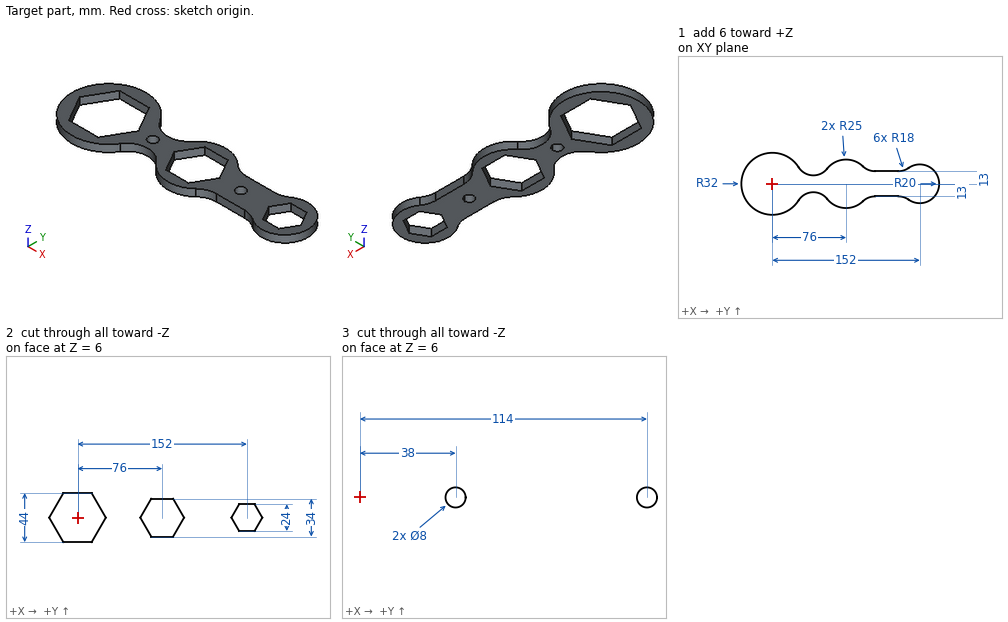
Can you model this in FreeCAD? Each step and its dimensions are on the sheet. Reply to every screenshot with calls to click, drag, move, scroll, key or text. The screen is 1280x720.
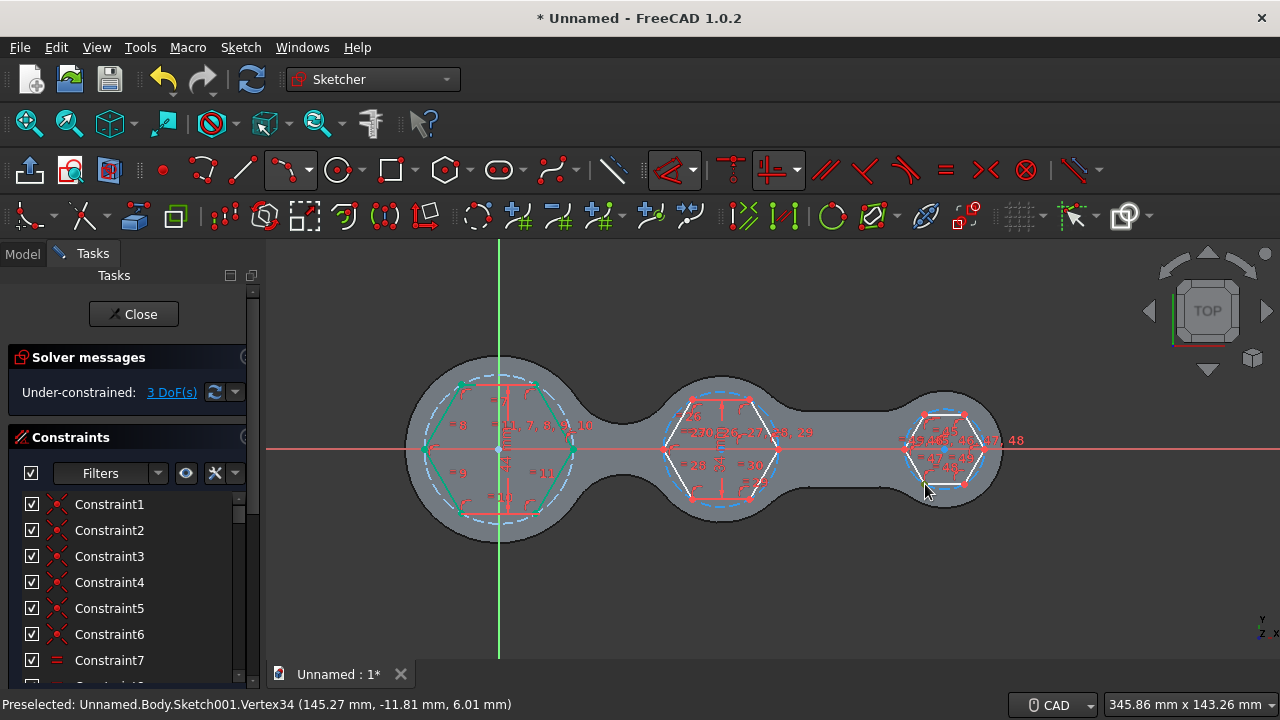
click(965, 415)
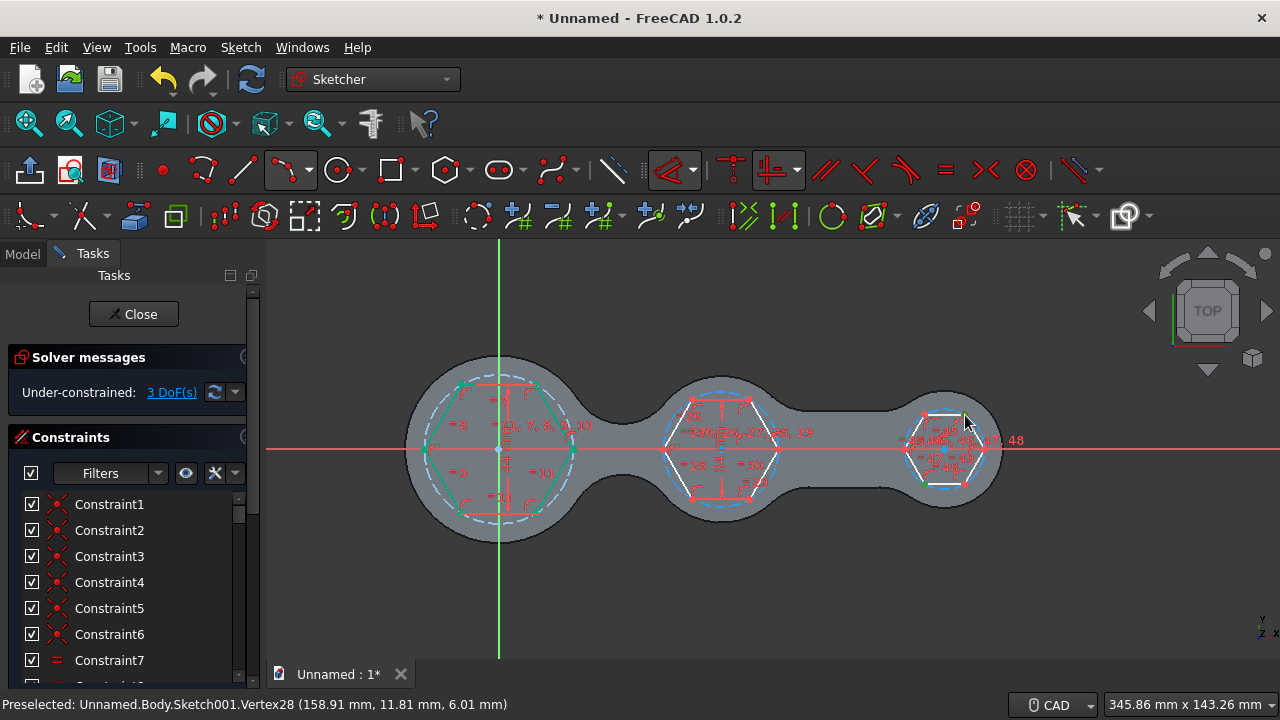
click(696, 170)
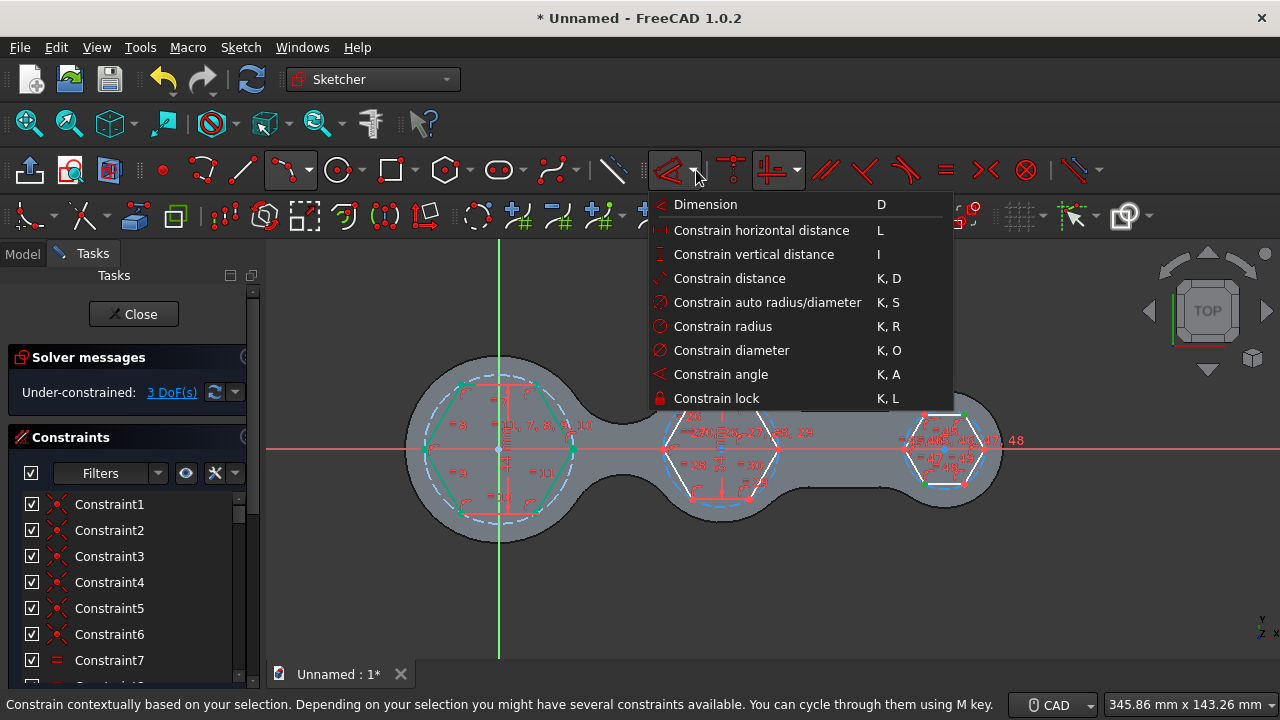
click(801, 254)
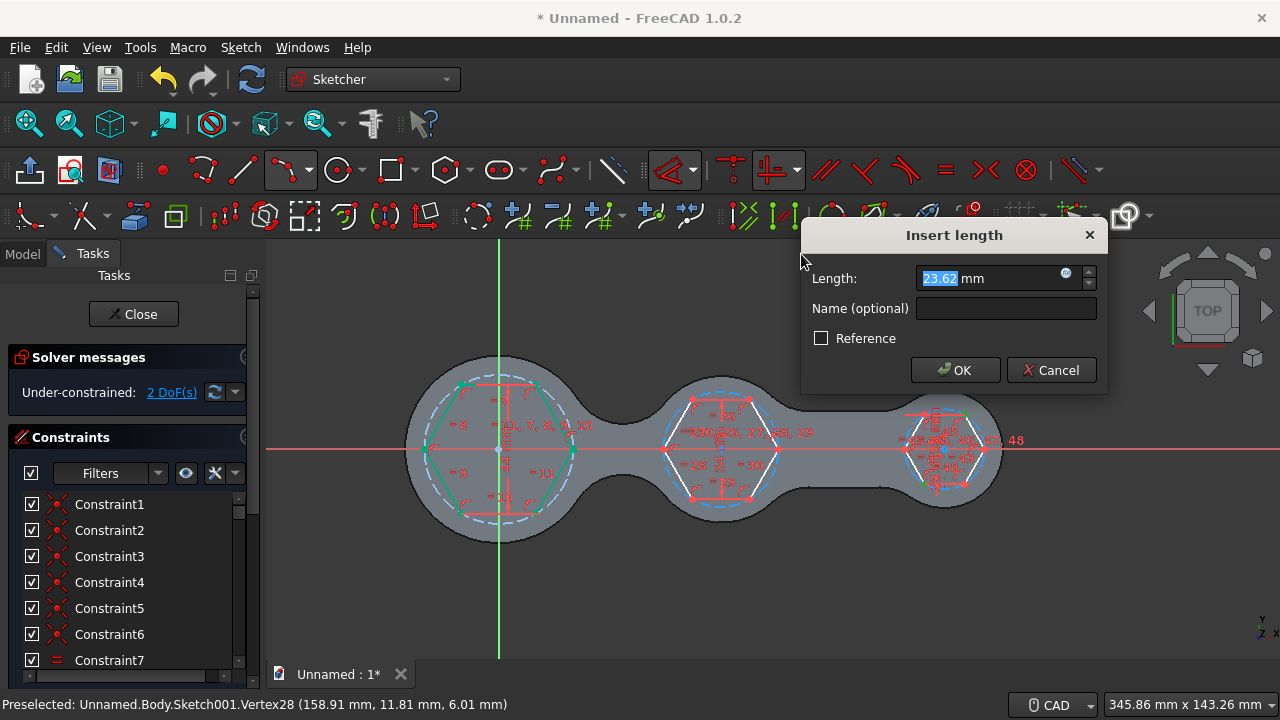
text(24)
key(Return)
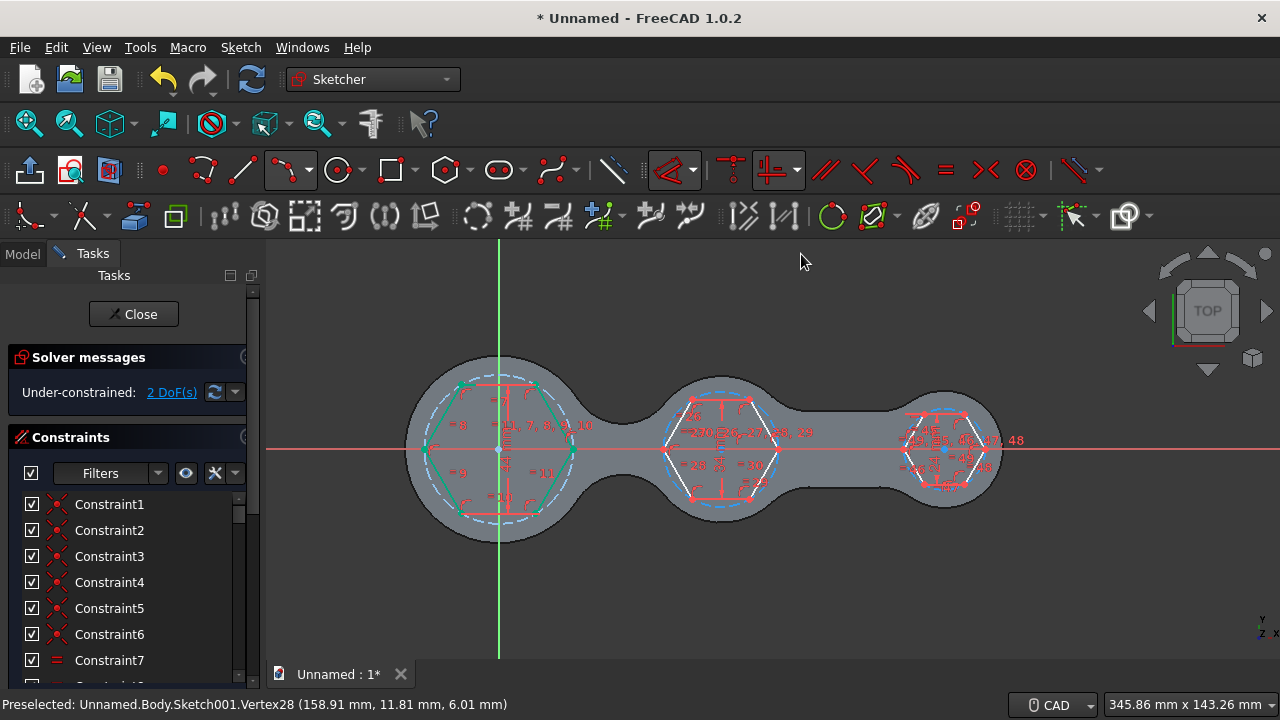
click(721, 449)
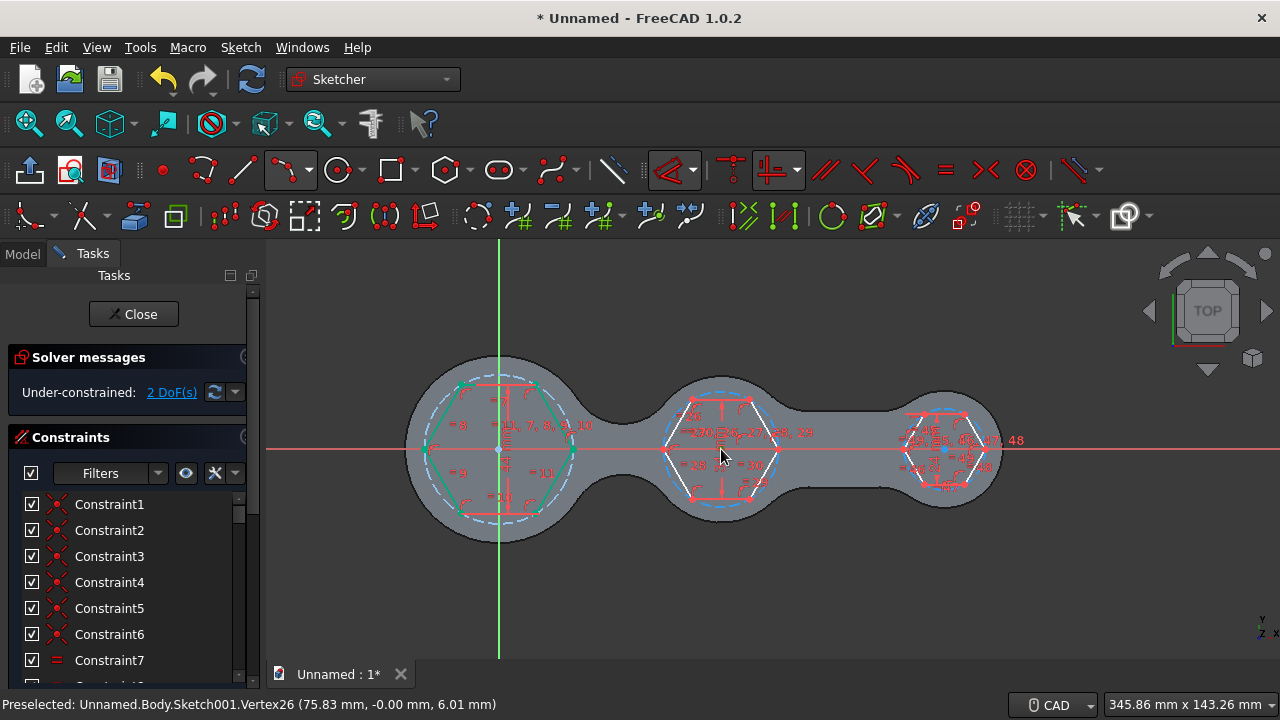
click(696, 170)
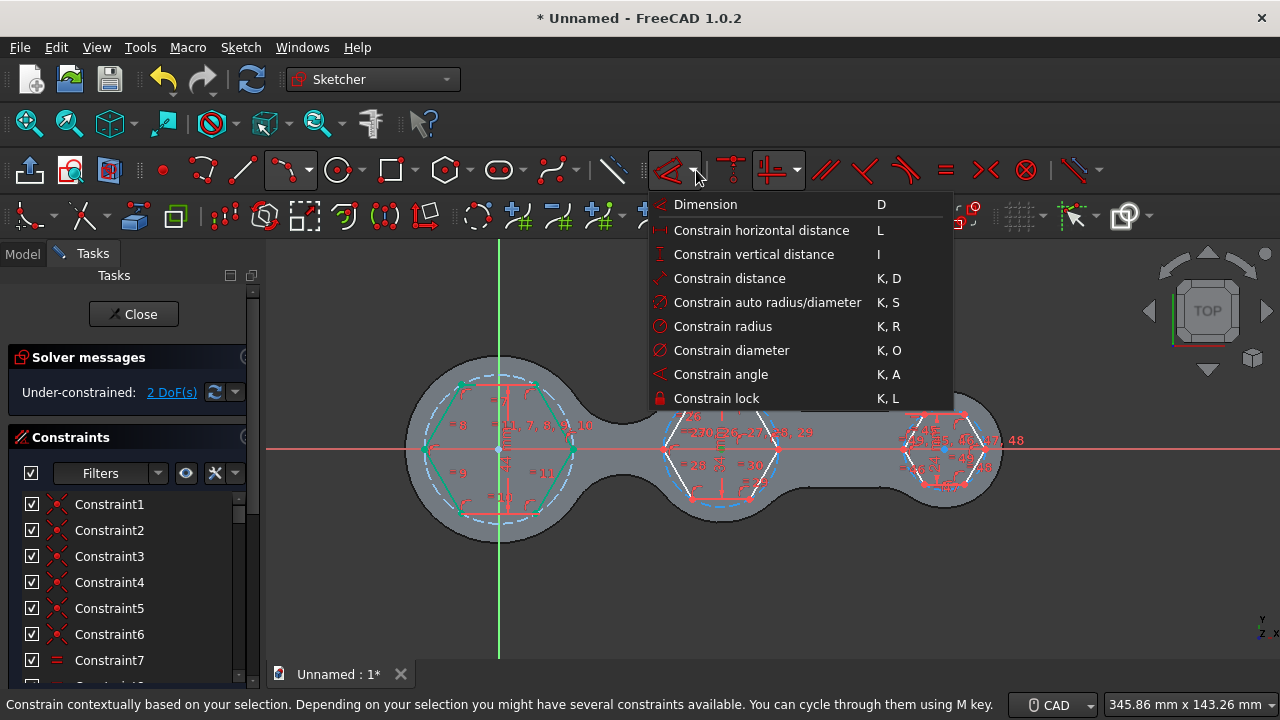
click(801, 230)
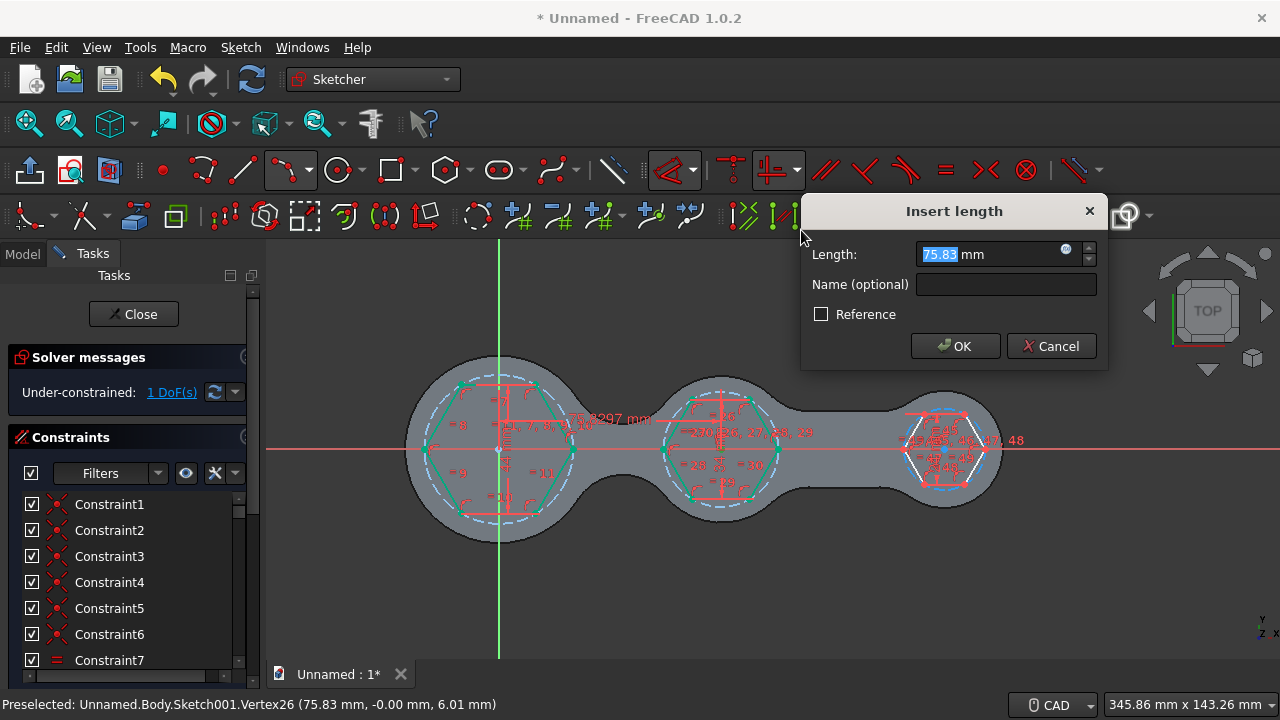
text(76)
key(Return)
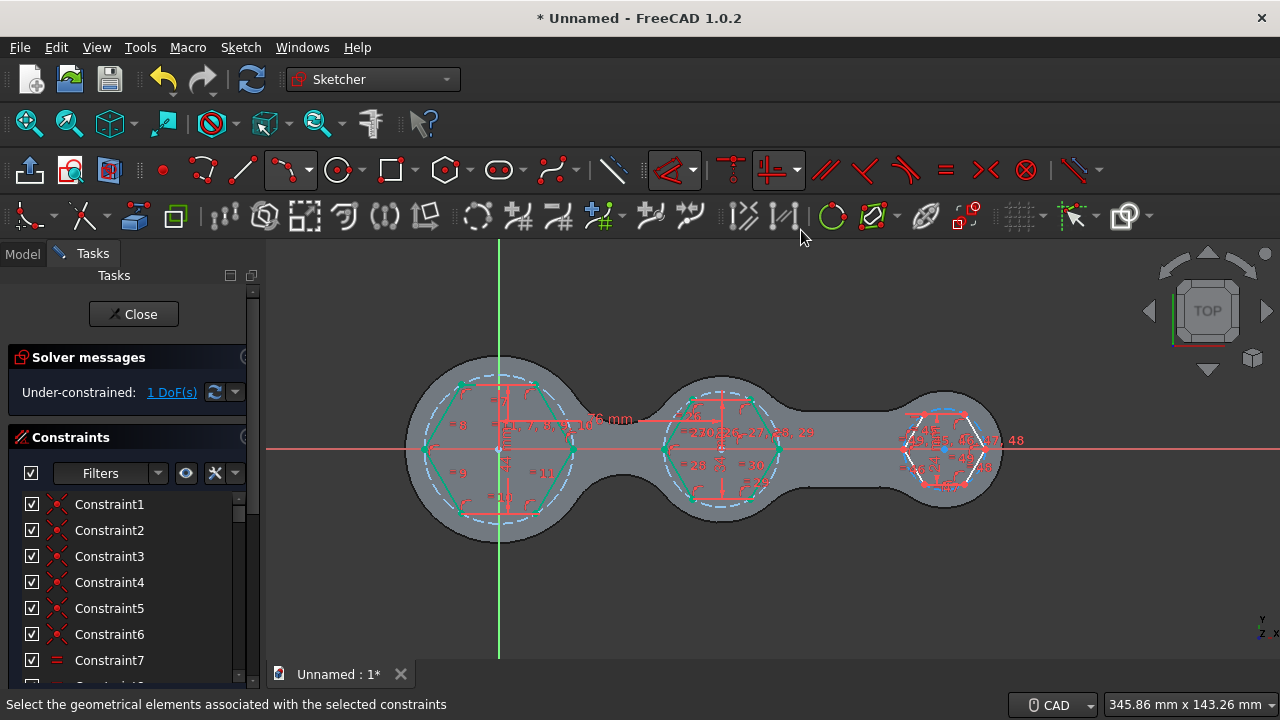
click(945, 449)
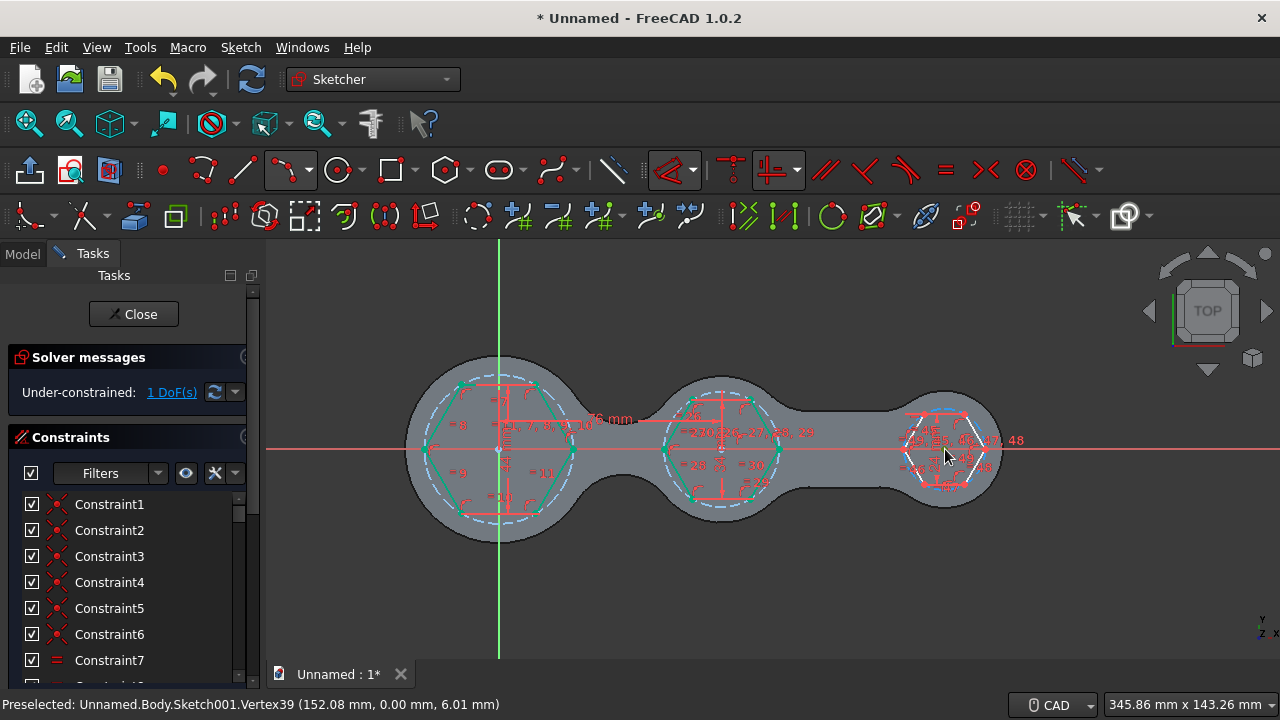
key(l)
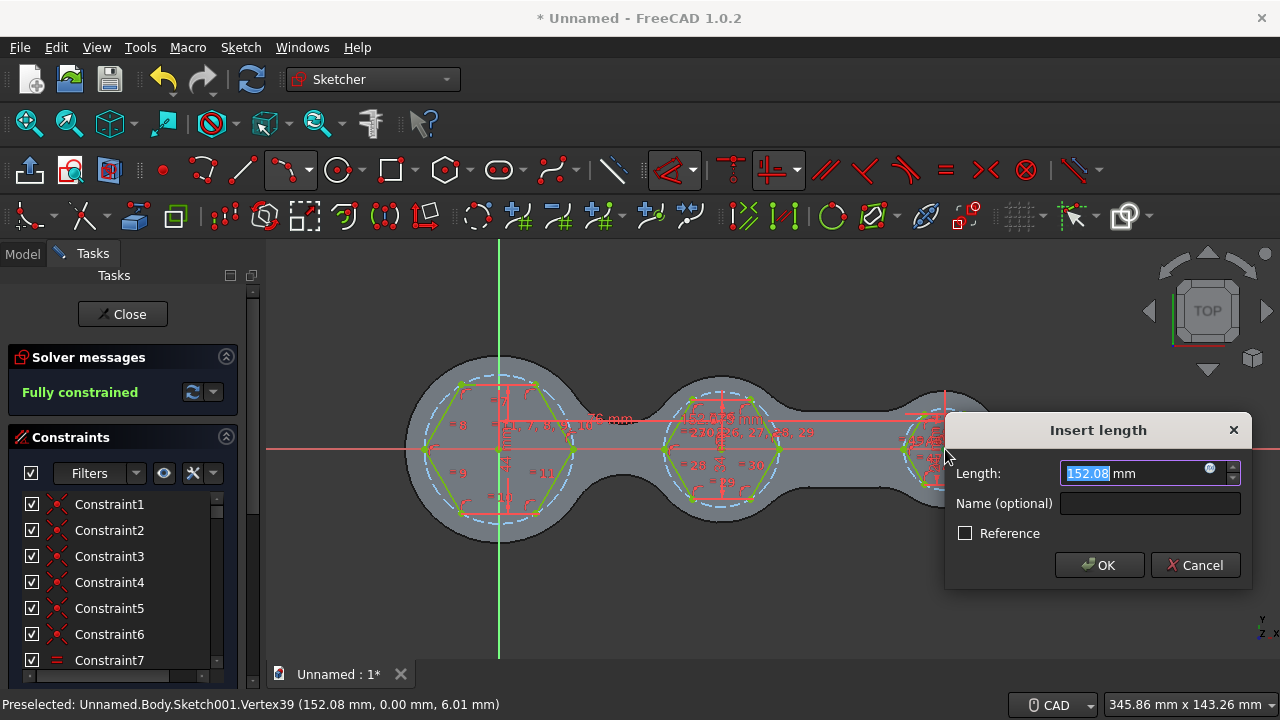
text(152)
key(Return)